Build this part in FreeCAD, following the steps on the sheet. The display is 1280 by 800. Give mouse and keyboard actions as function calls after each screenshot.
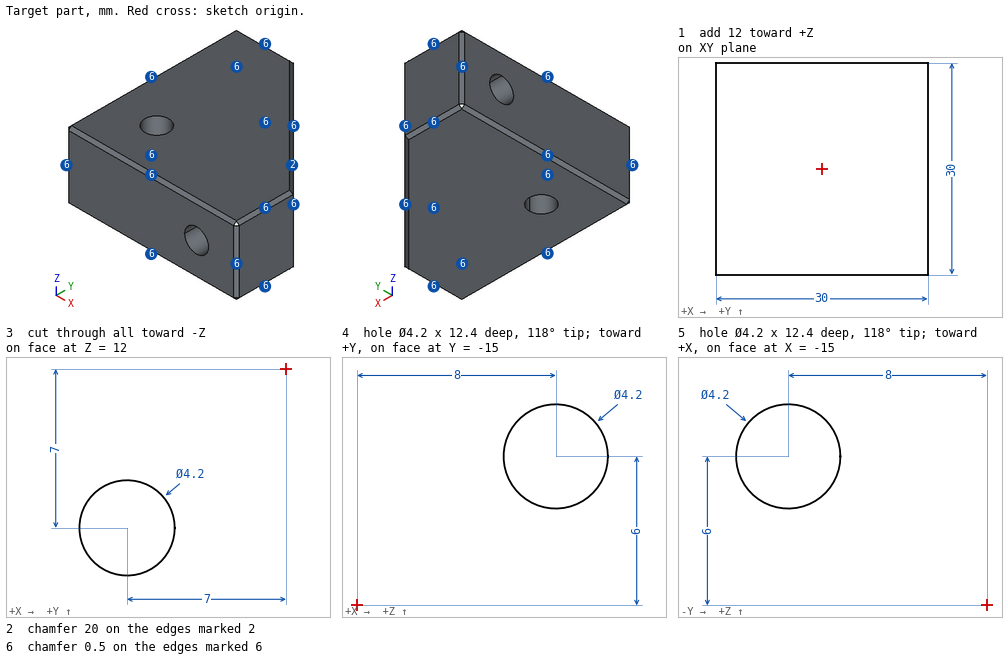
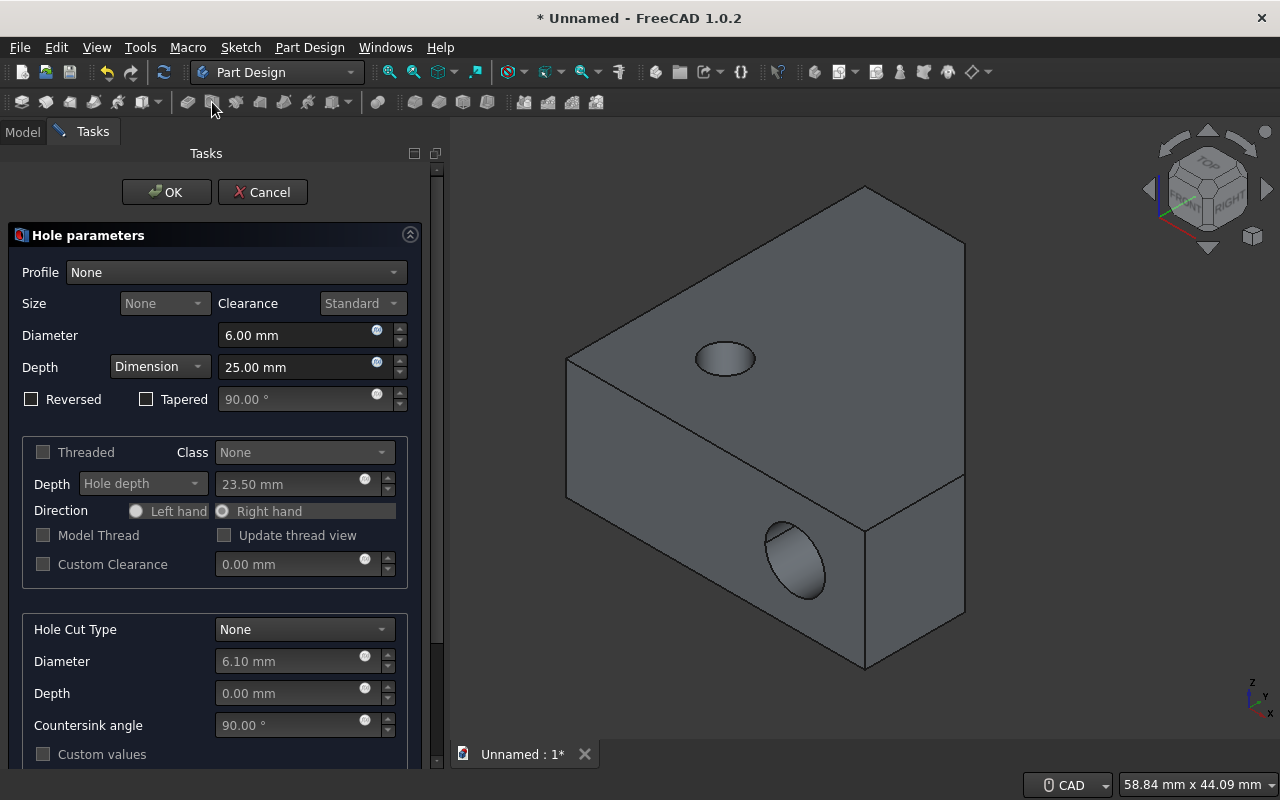
triple_click(305, 335)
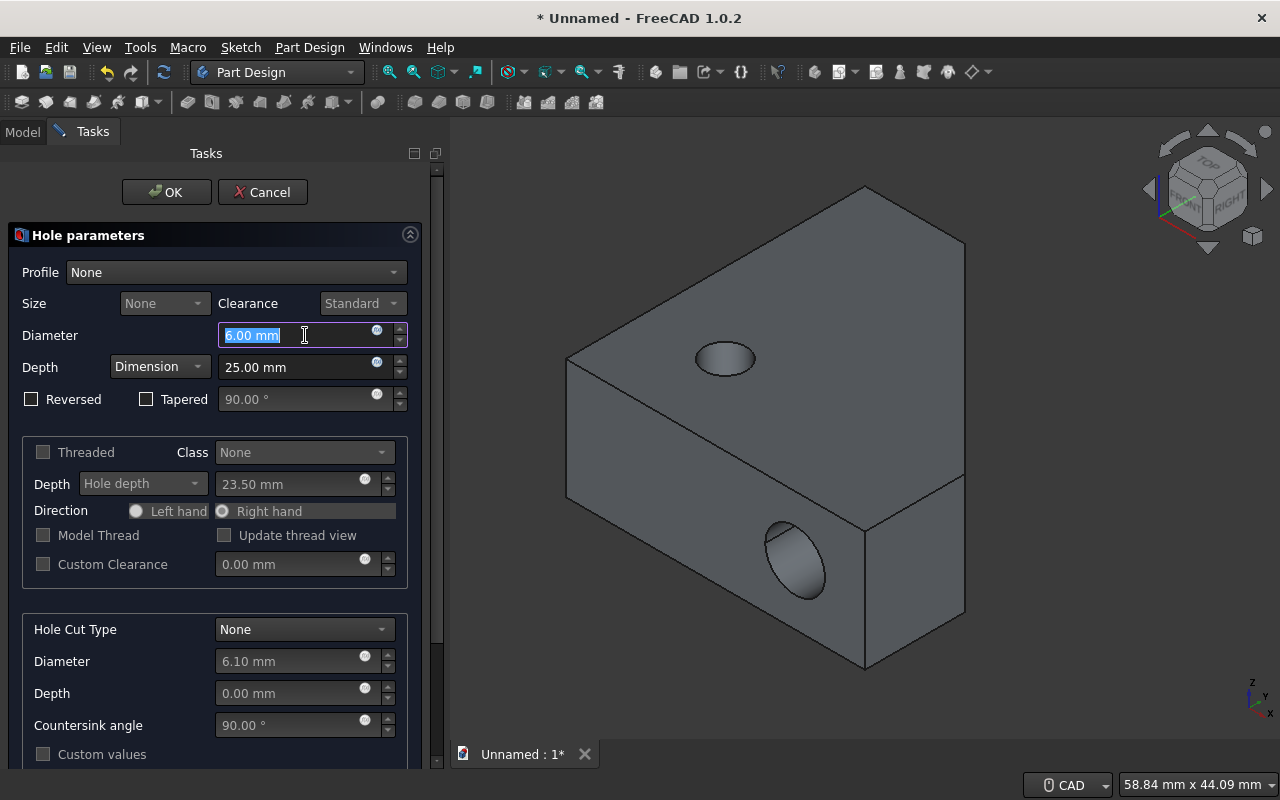
text(4.2)
key(Tab)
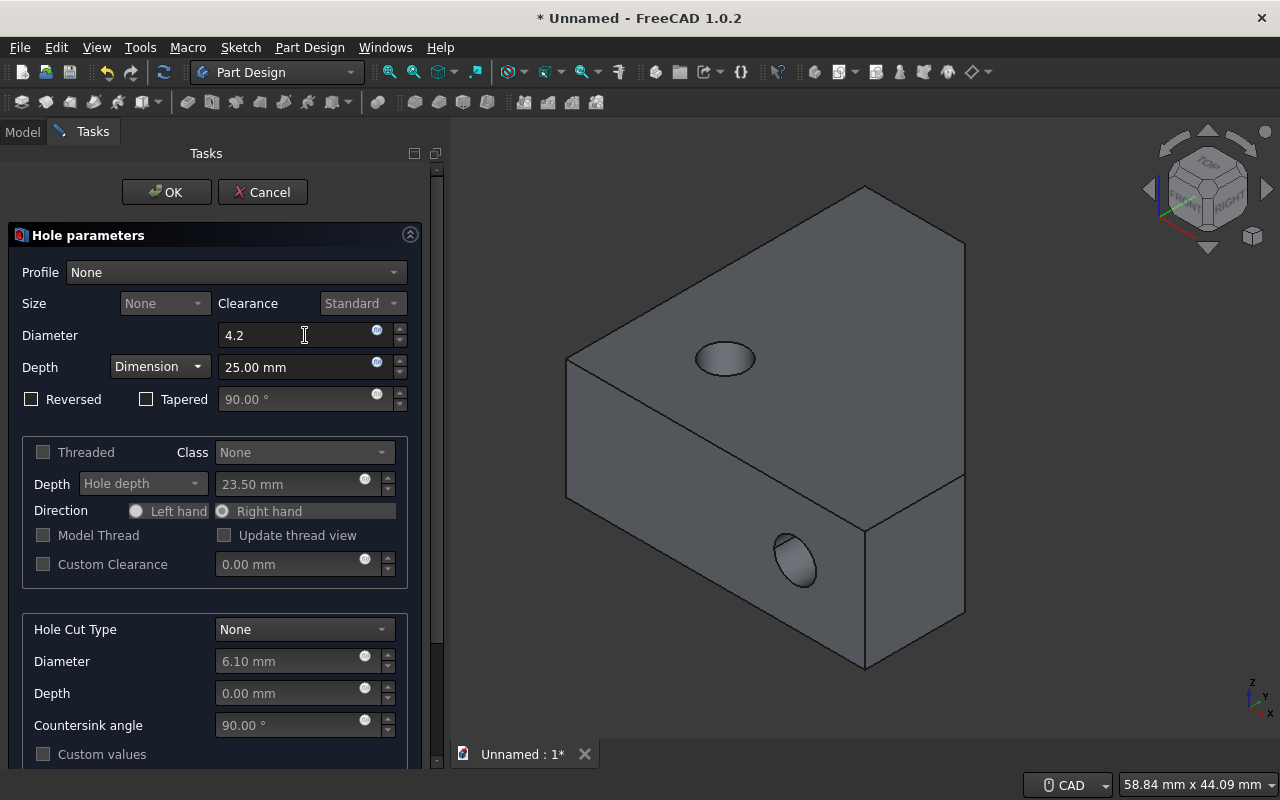
triple_click(305, 367)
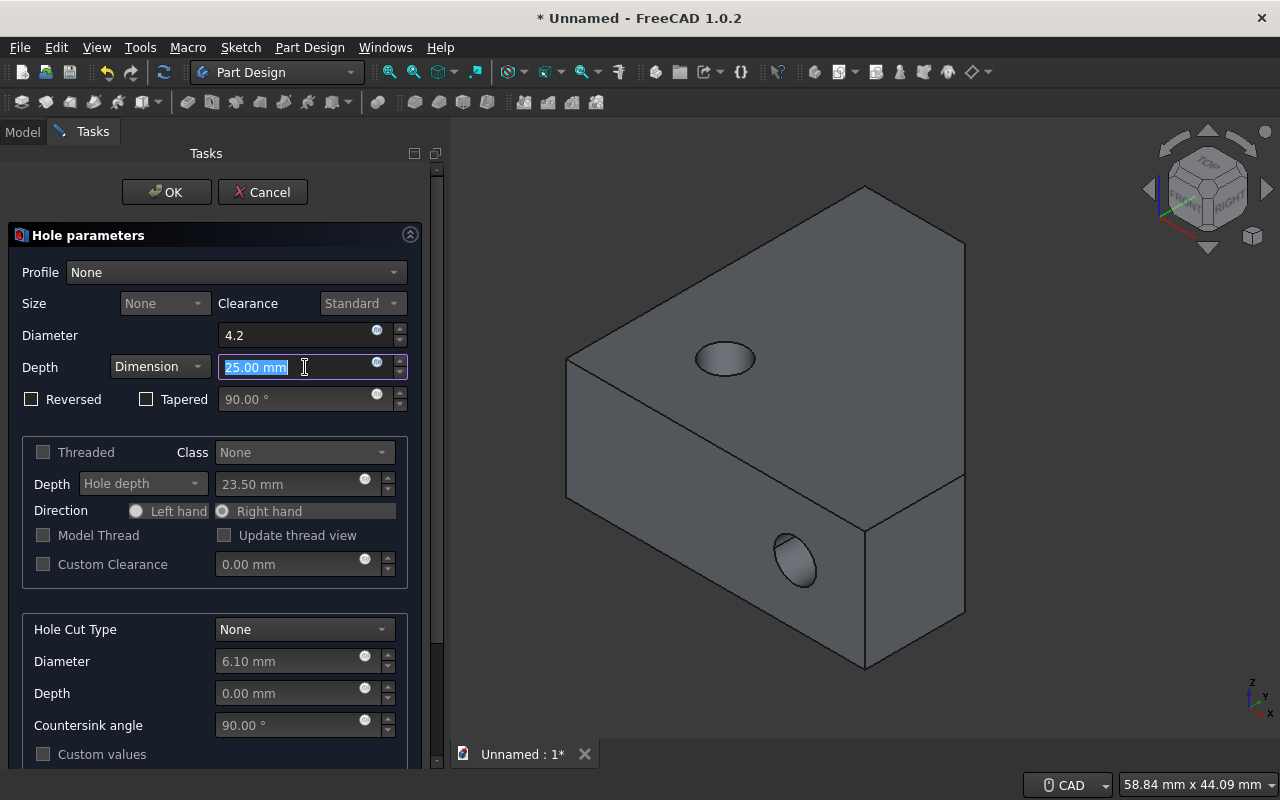
text(12.4)
key(Tab)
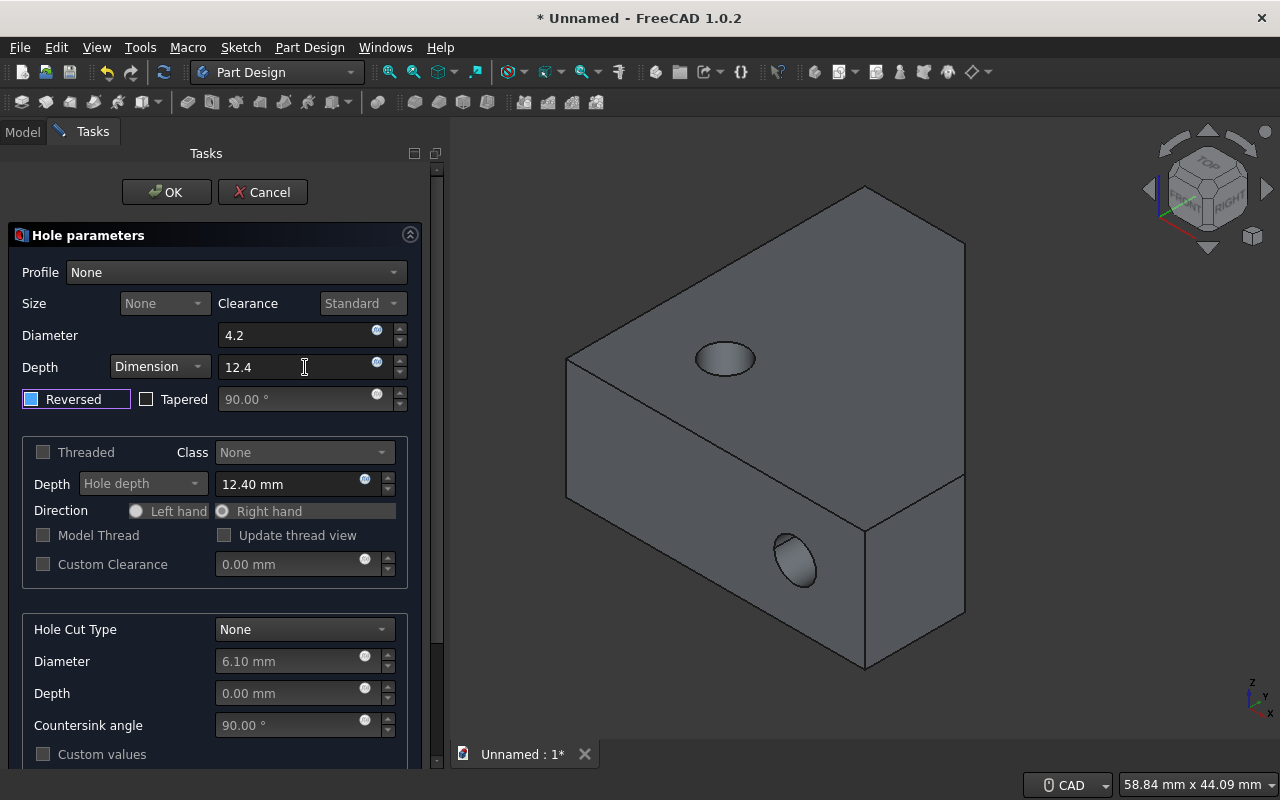
click(167, 192)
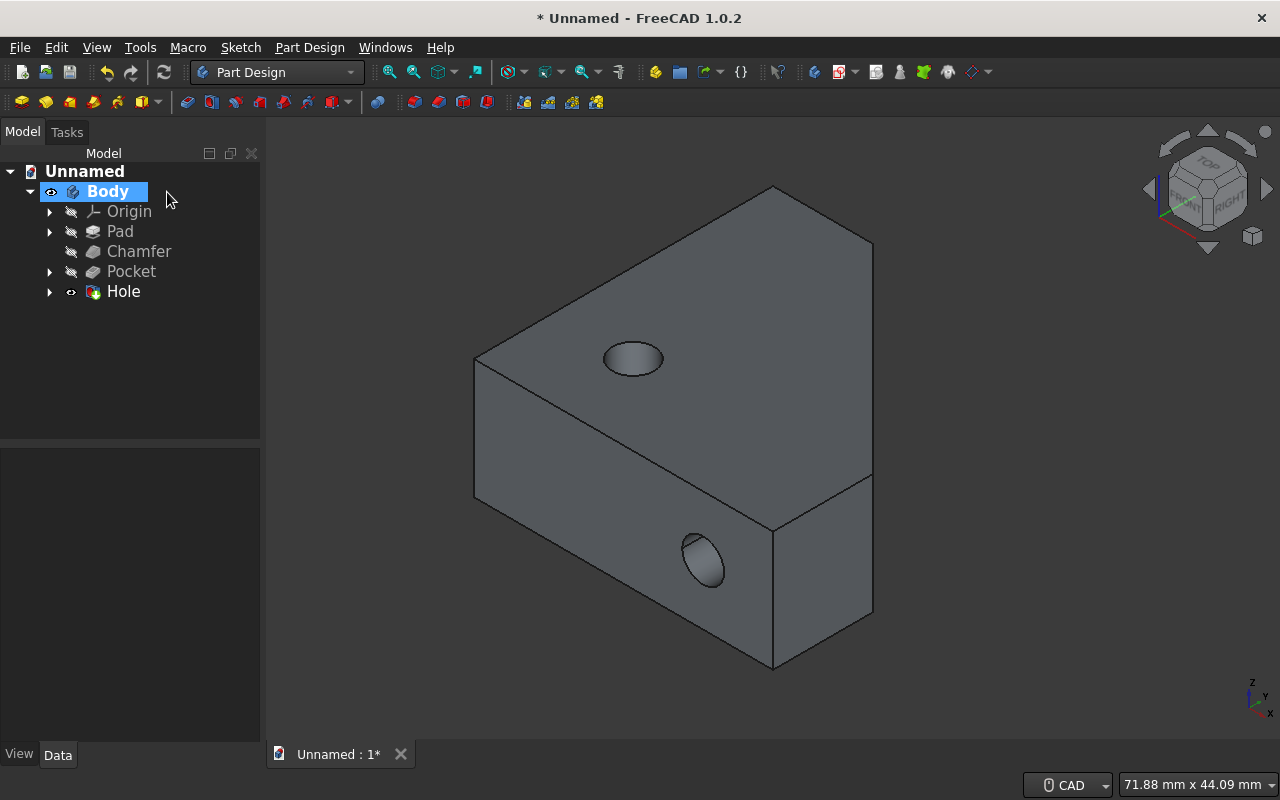
key(6)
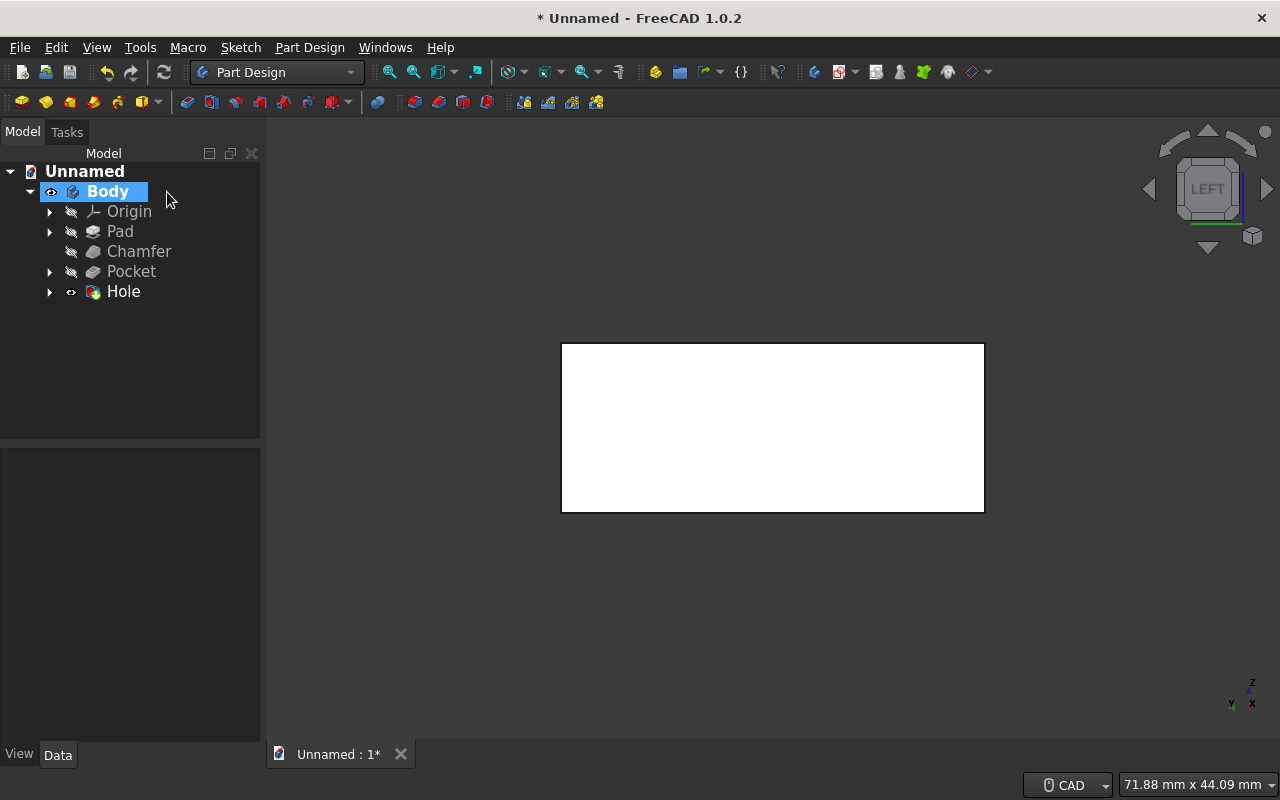
key(v)
key(f)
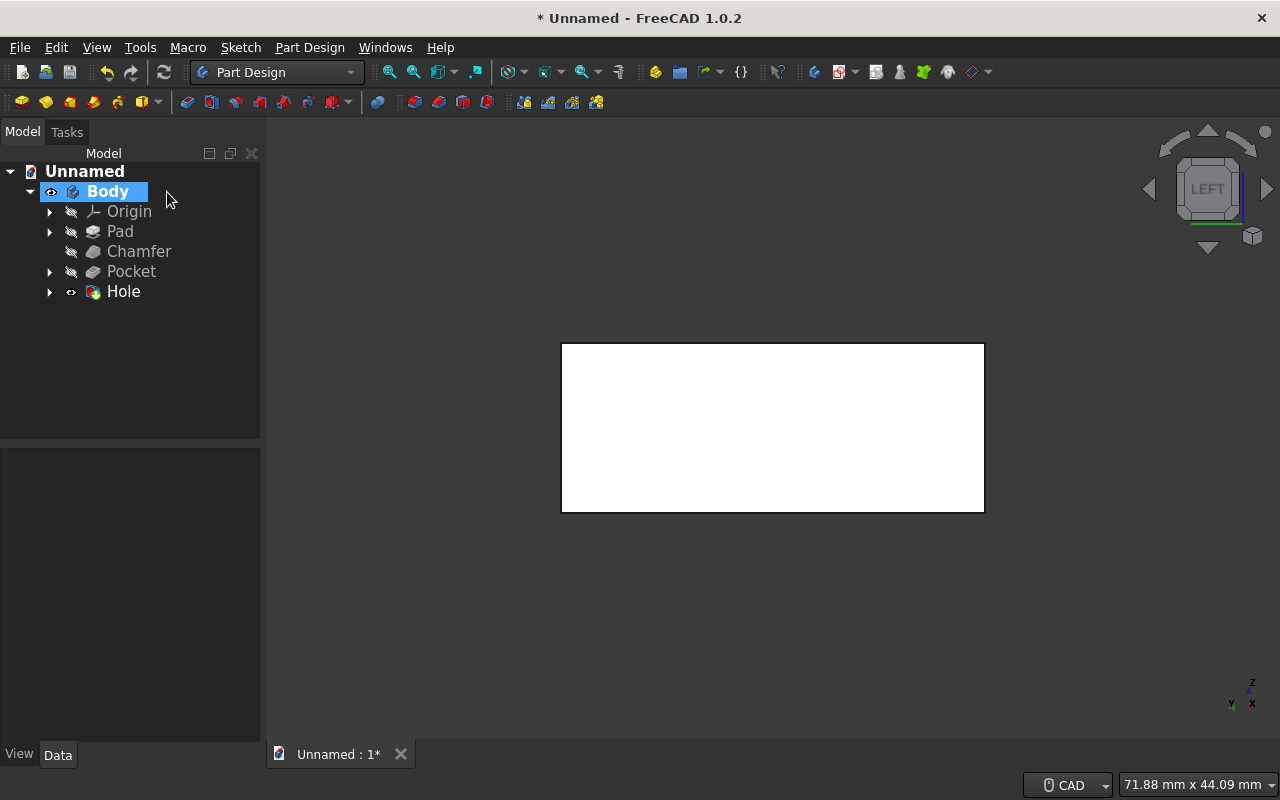
click(652, 427)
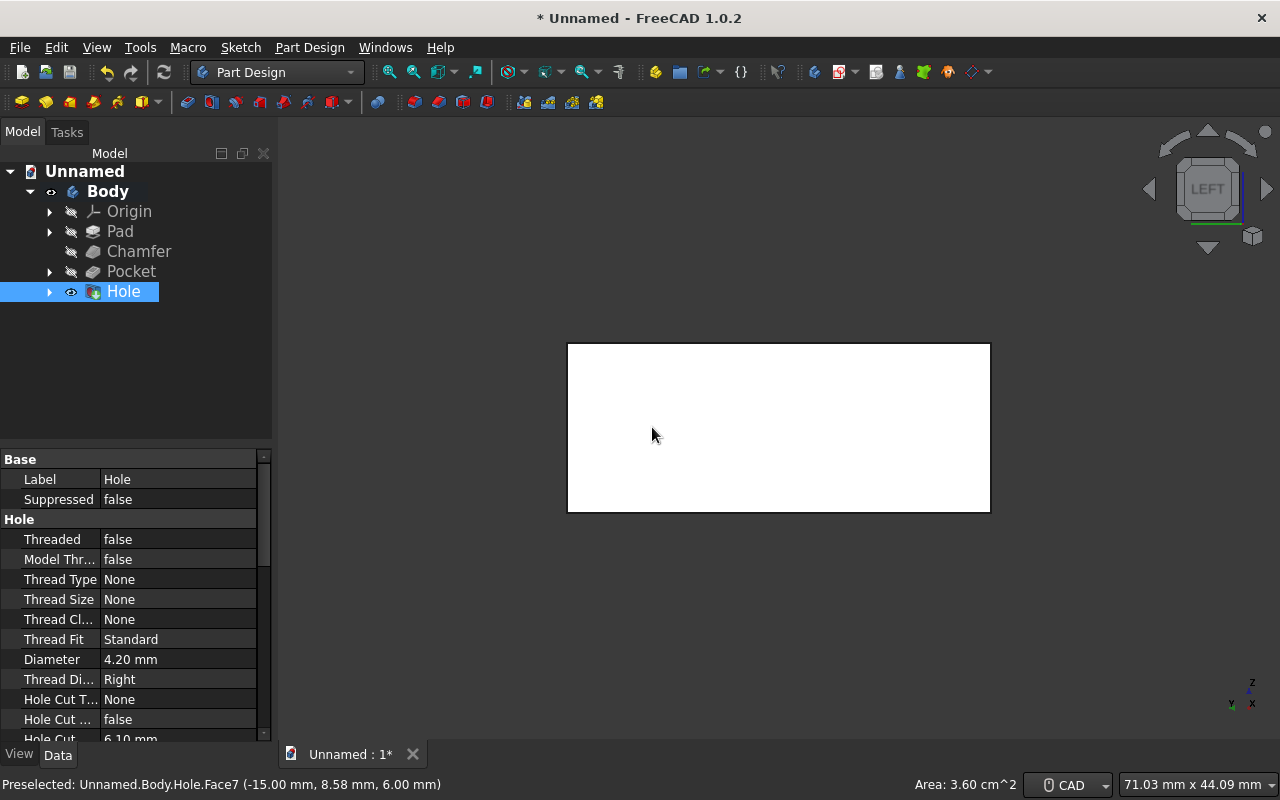
click(840, 72)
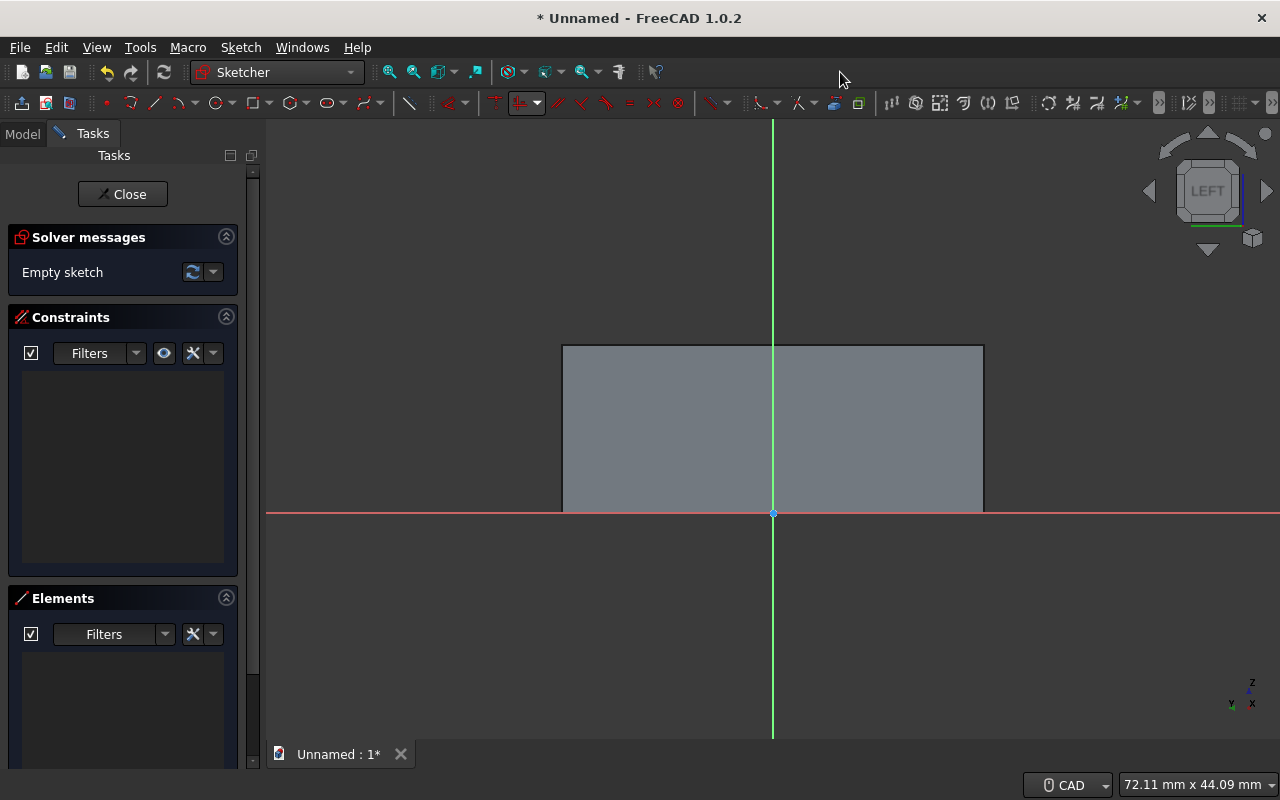
scroll(701, 468, up, 6)